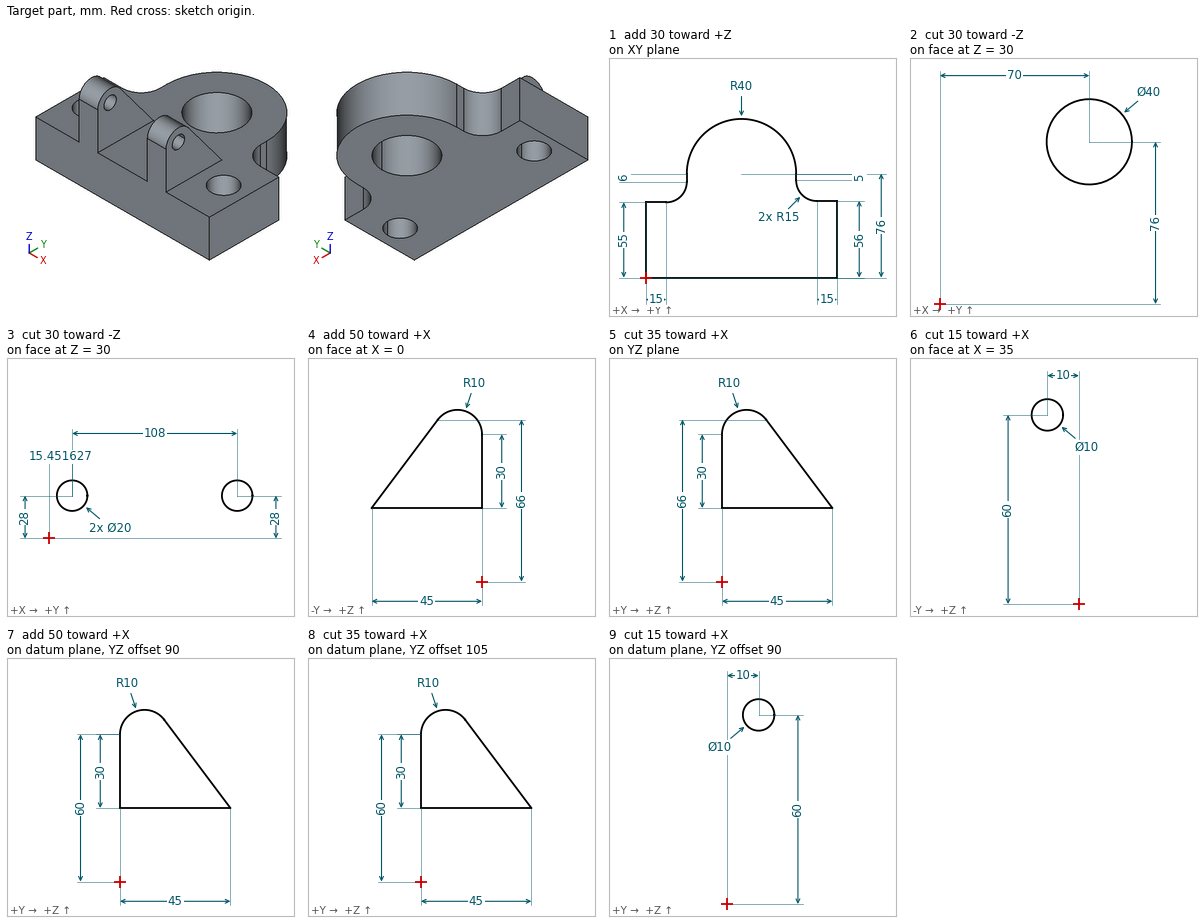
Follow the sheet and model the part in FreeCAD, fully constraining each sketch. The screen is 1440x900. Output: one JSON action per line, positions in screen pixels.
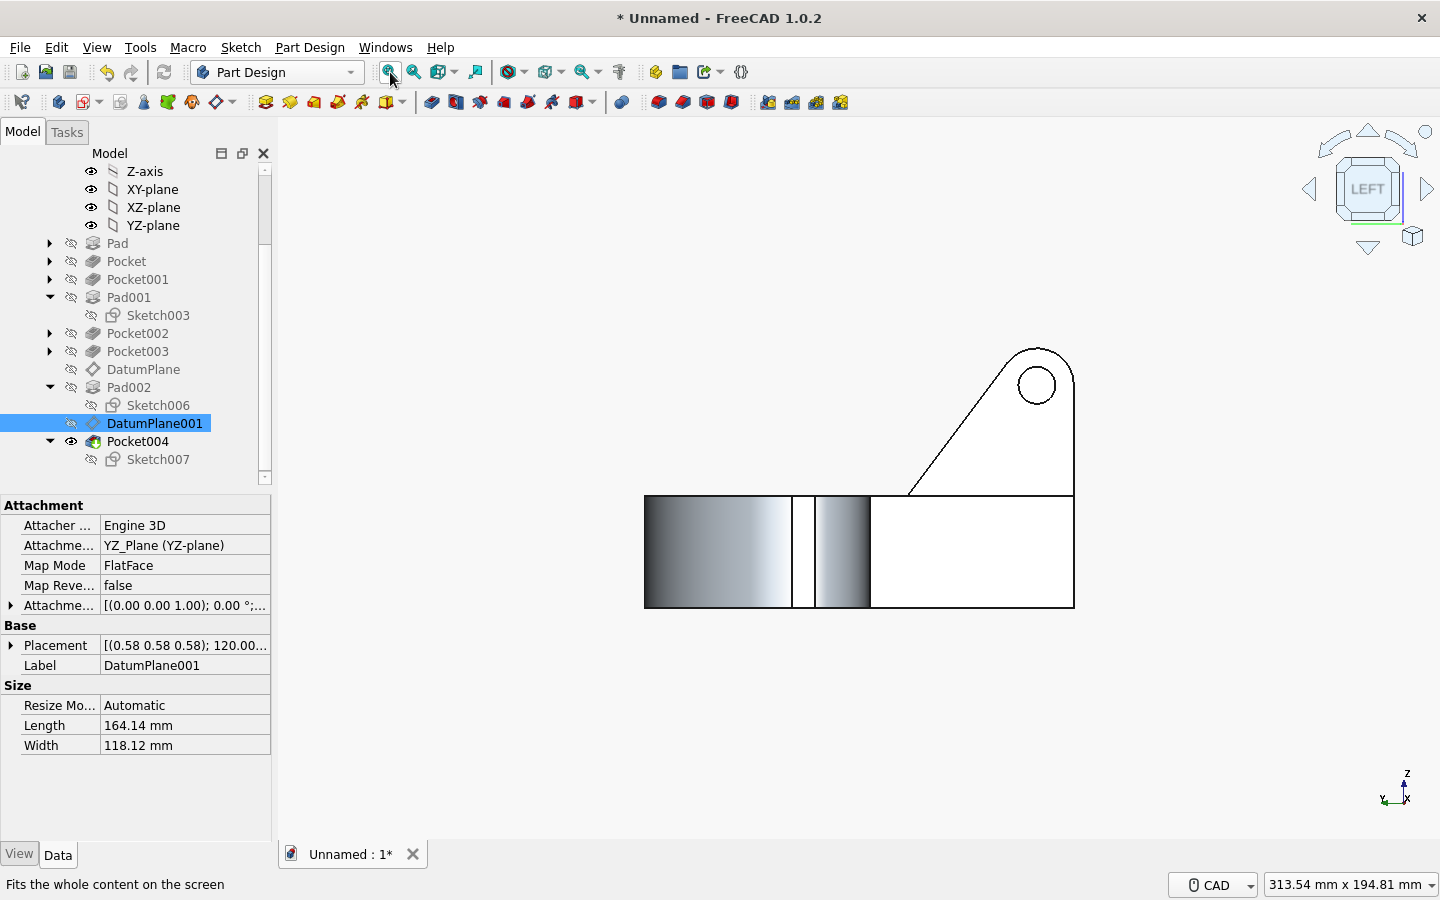
{"action": "key", "text": "1"}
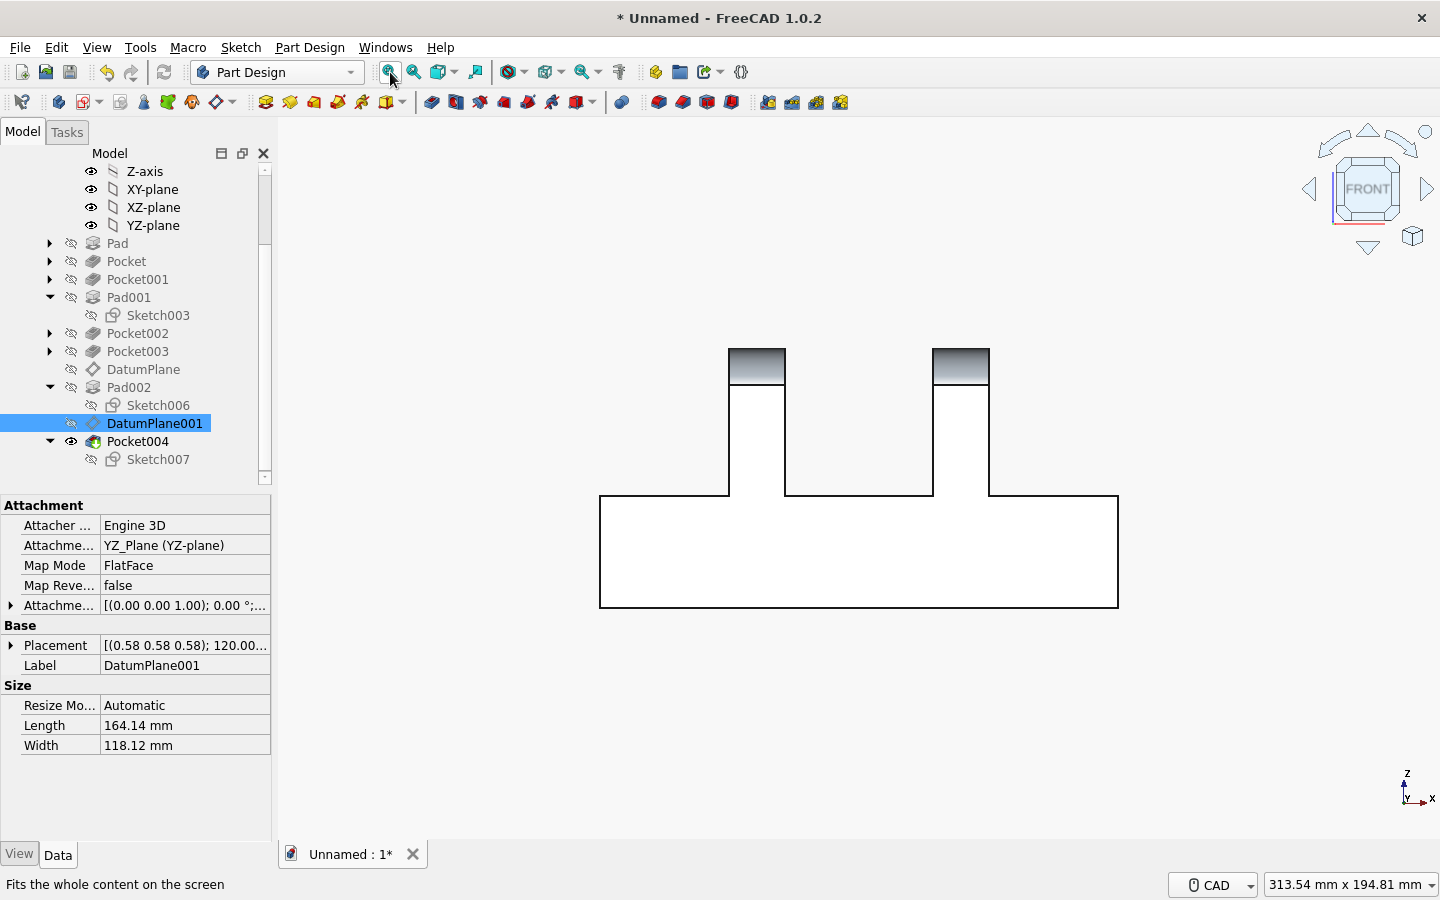
{"action": "key", "text": "v f"}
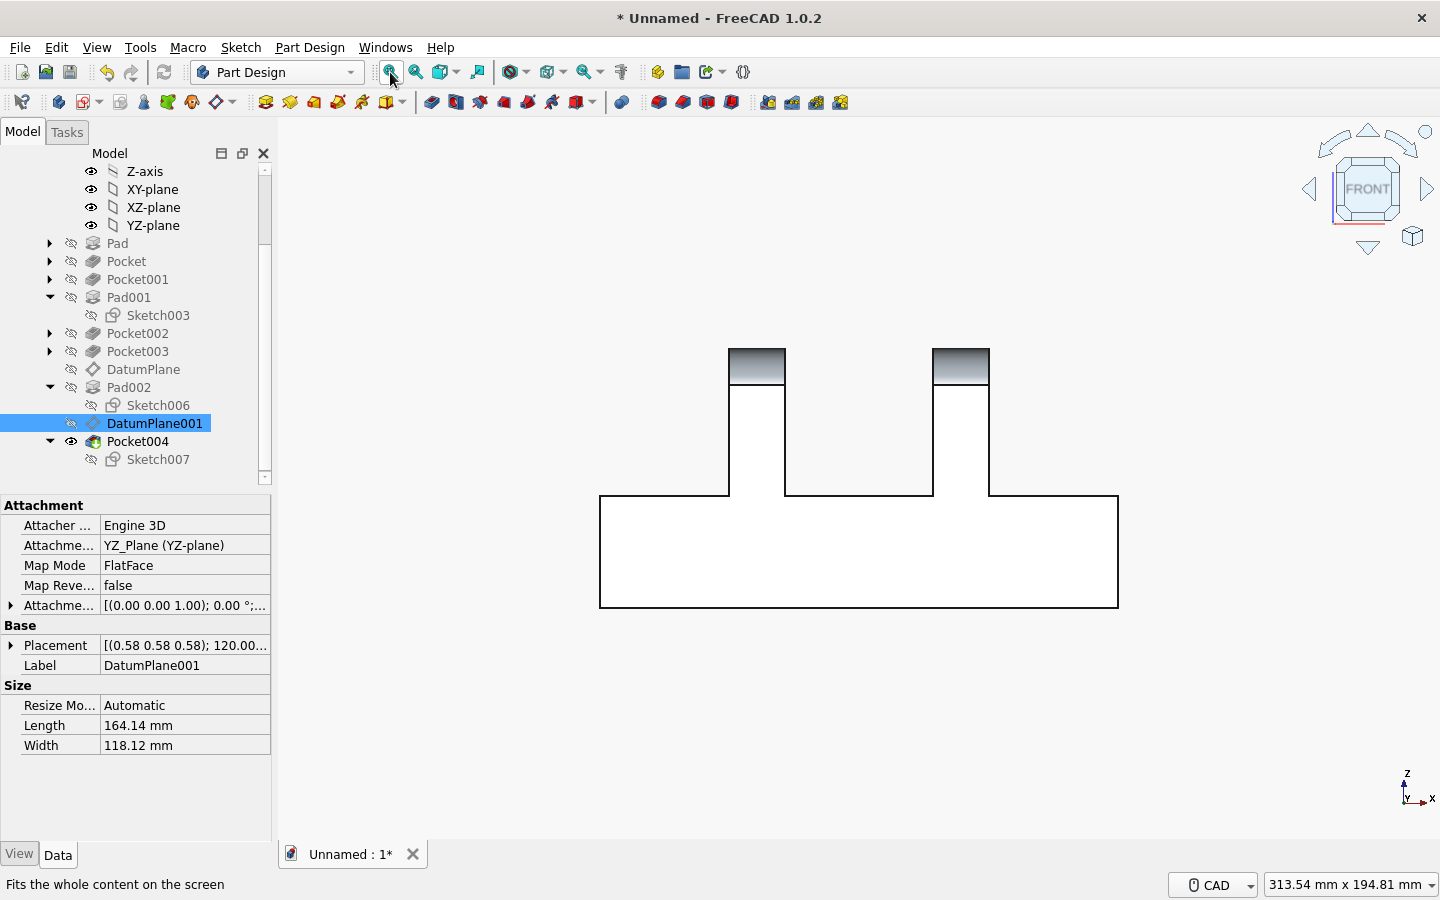
{"action": "scroll", "coordinate": [160, 311], "scroll_direction": "down", "scroll_amount": 3}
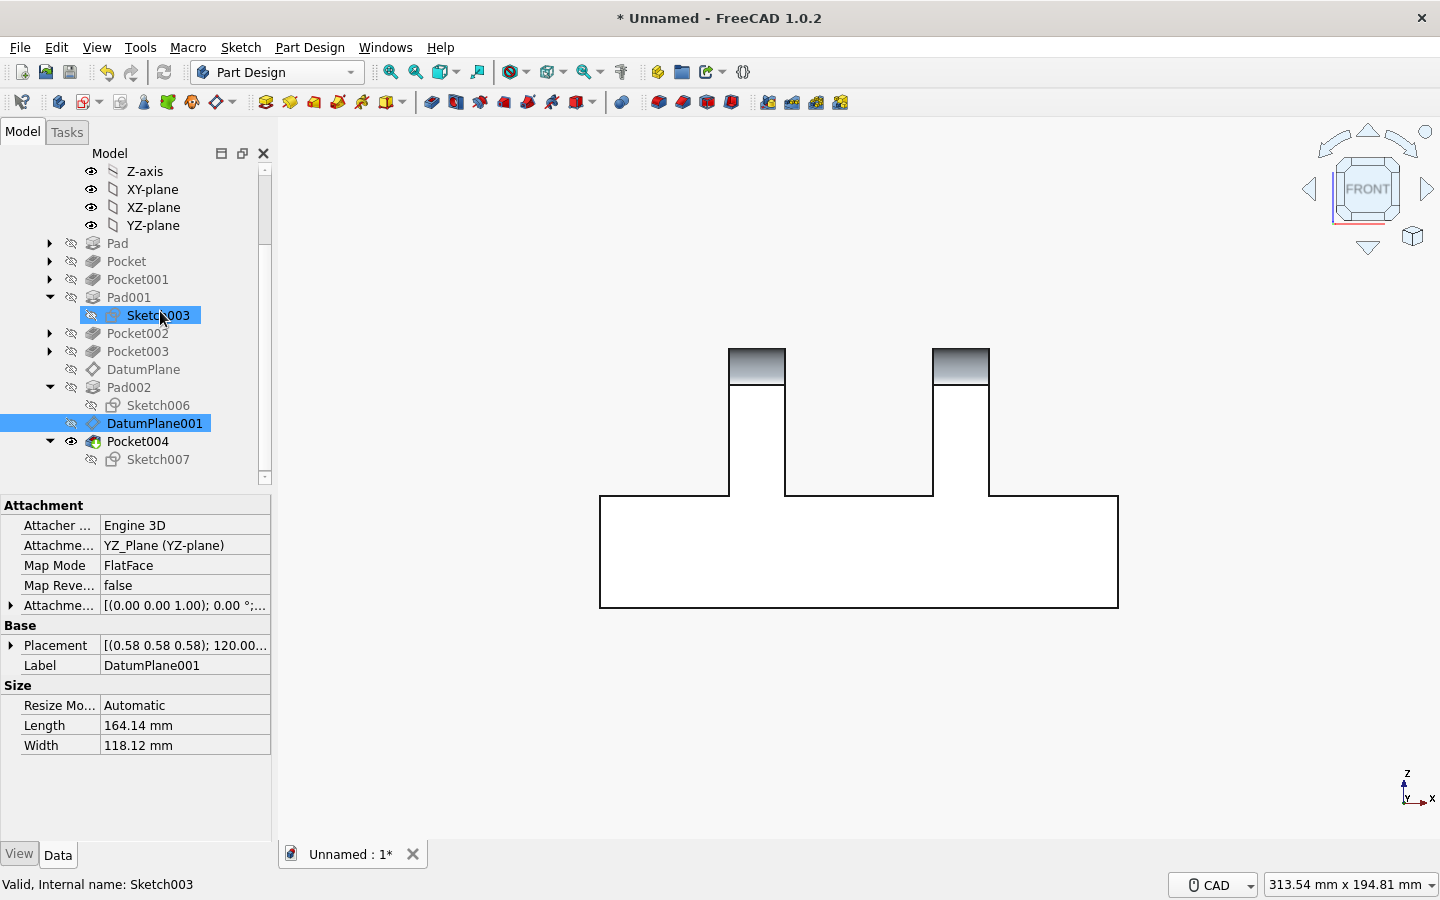
{"action": "scroll", "coordinate": [160, 311], "scroll_direction": "up", "scroll_amount": 15}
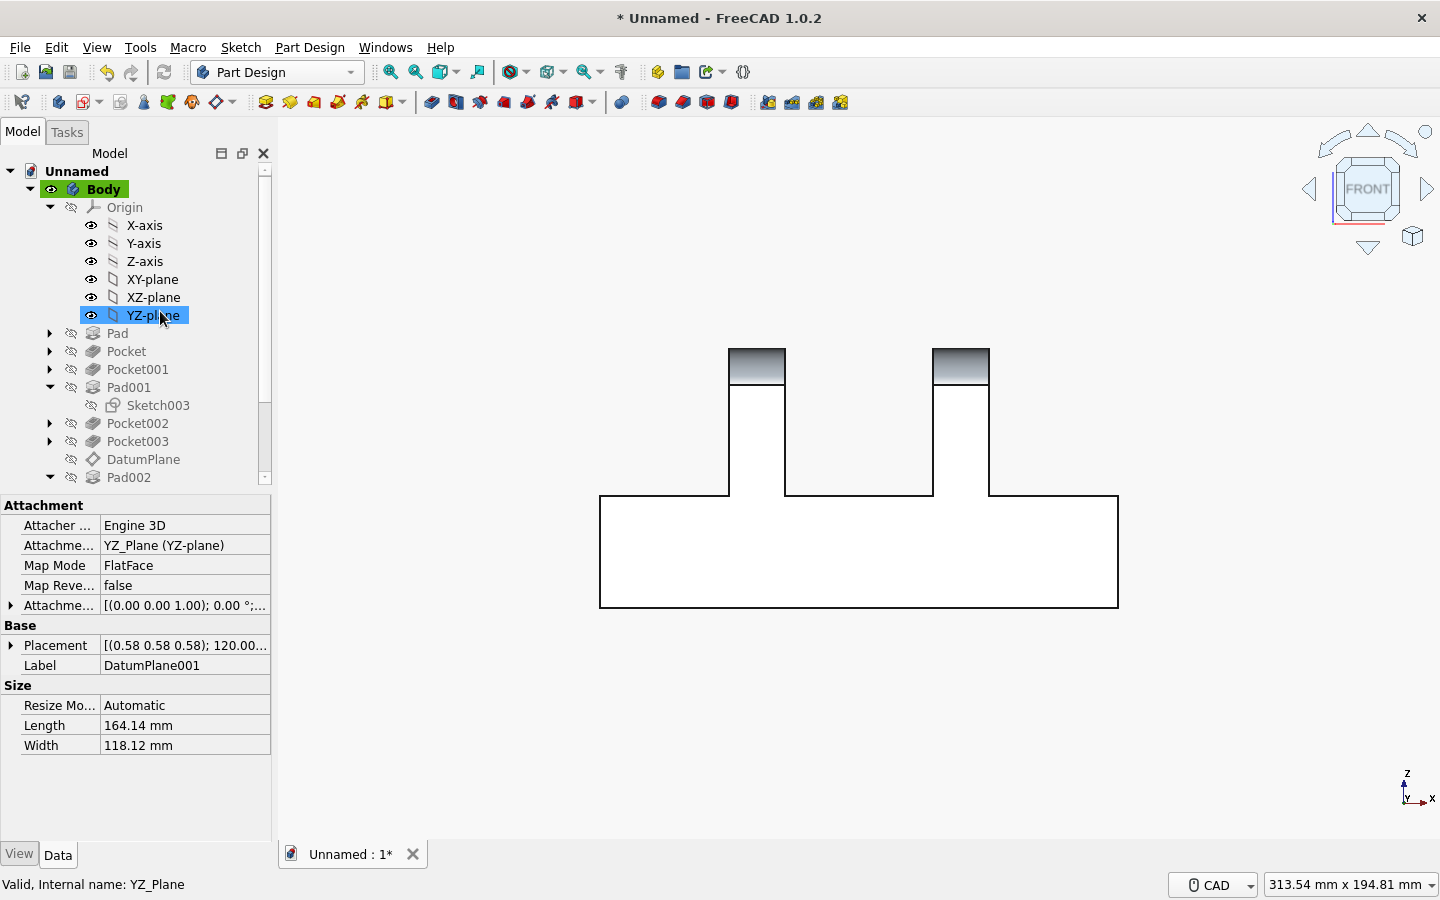
{"action": "left_click", "coordinate": [136, 315]}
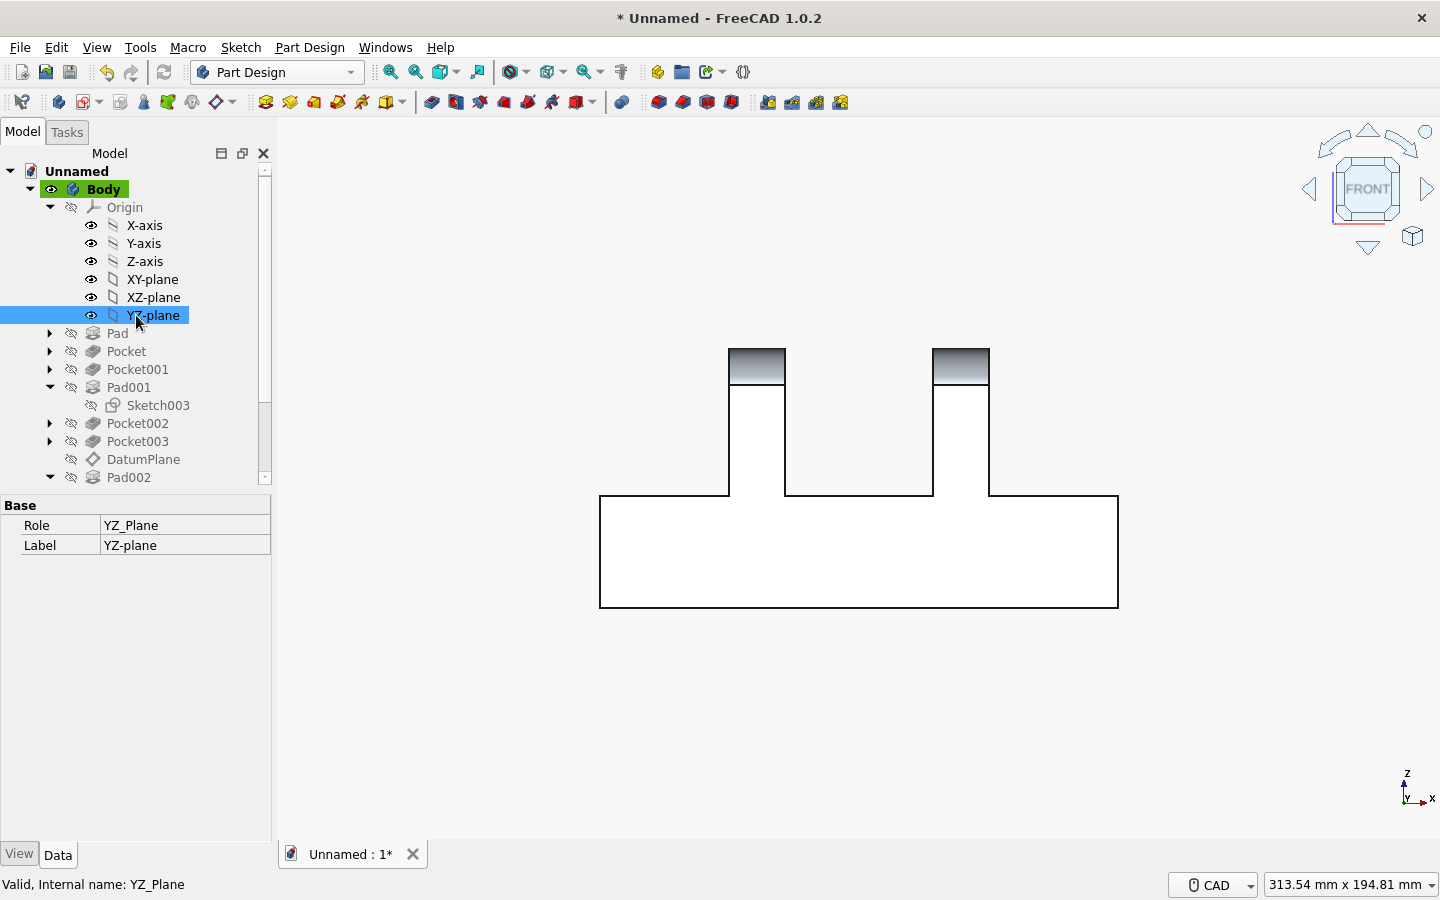
{"action": "left_click", "coordinate": [216, 102]}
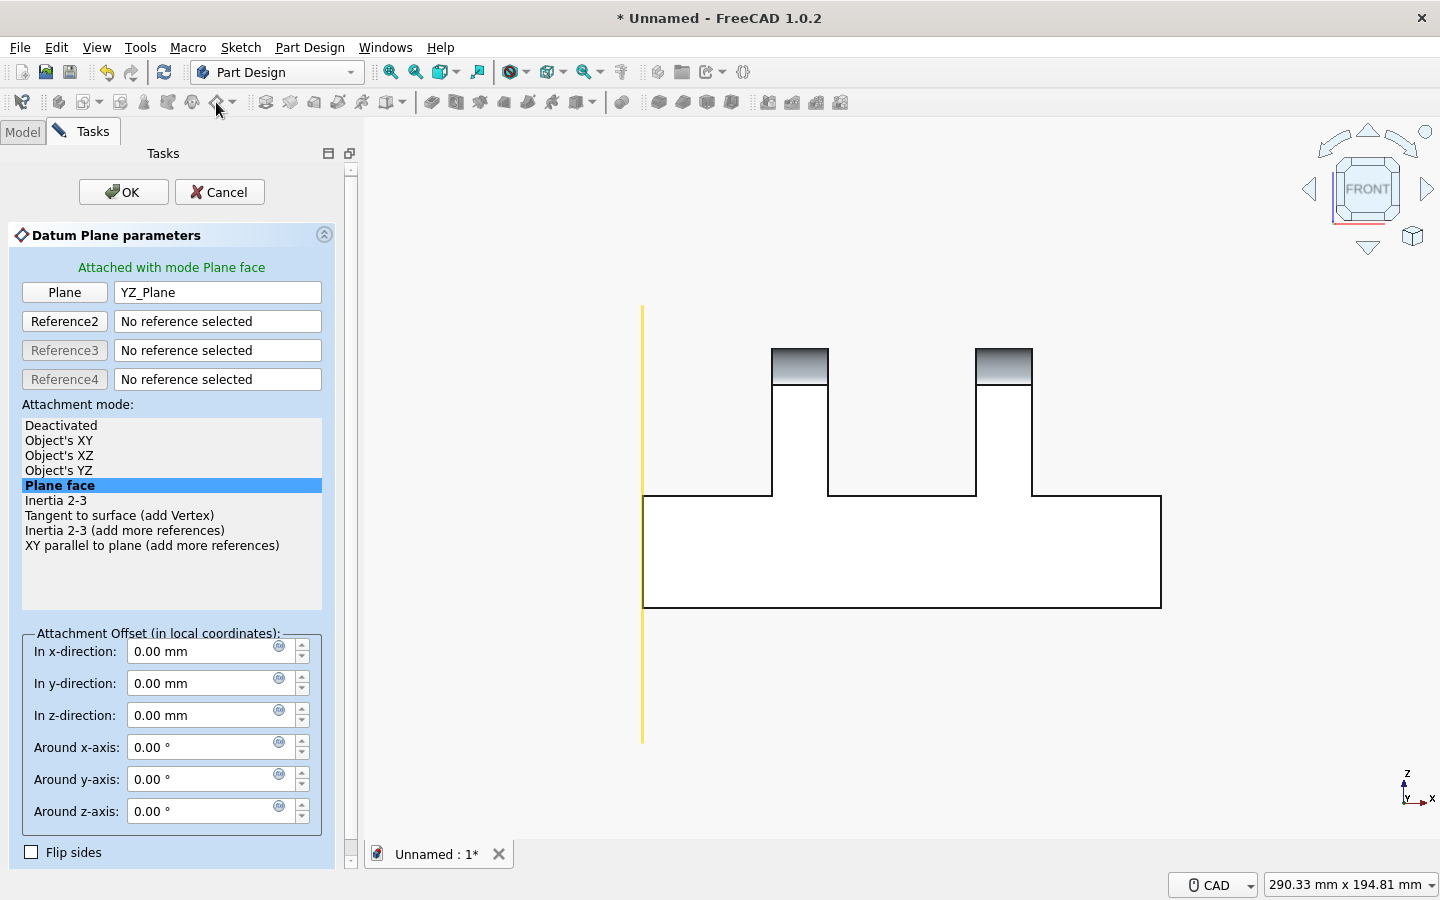
{"action": "triple_click", "coordinate": [210, 715]}